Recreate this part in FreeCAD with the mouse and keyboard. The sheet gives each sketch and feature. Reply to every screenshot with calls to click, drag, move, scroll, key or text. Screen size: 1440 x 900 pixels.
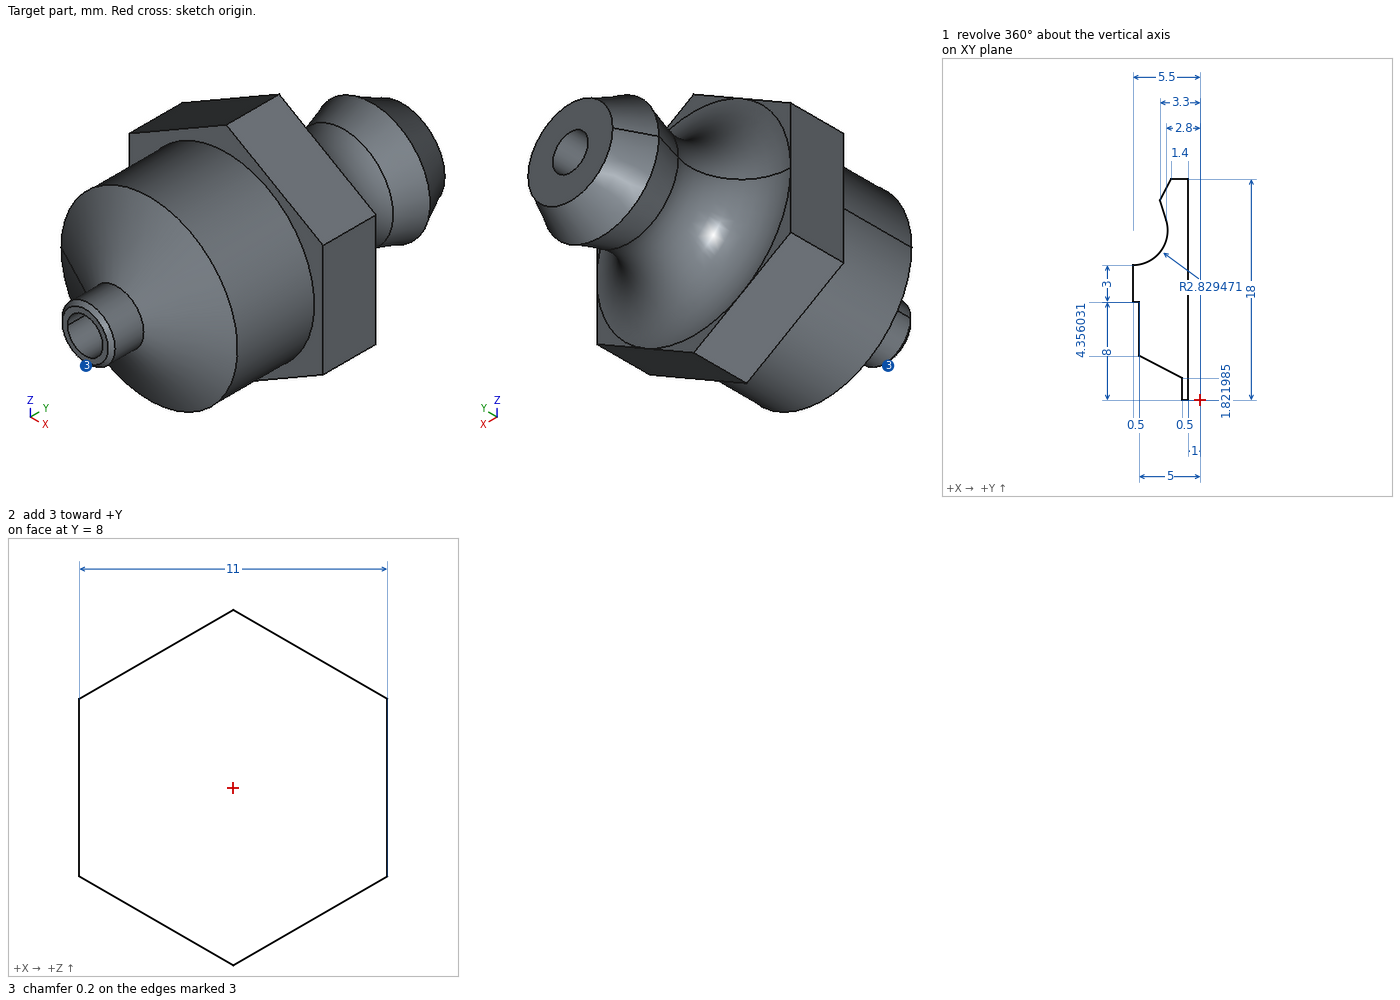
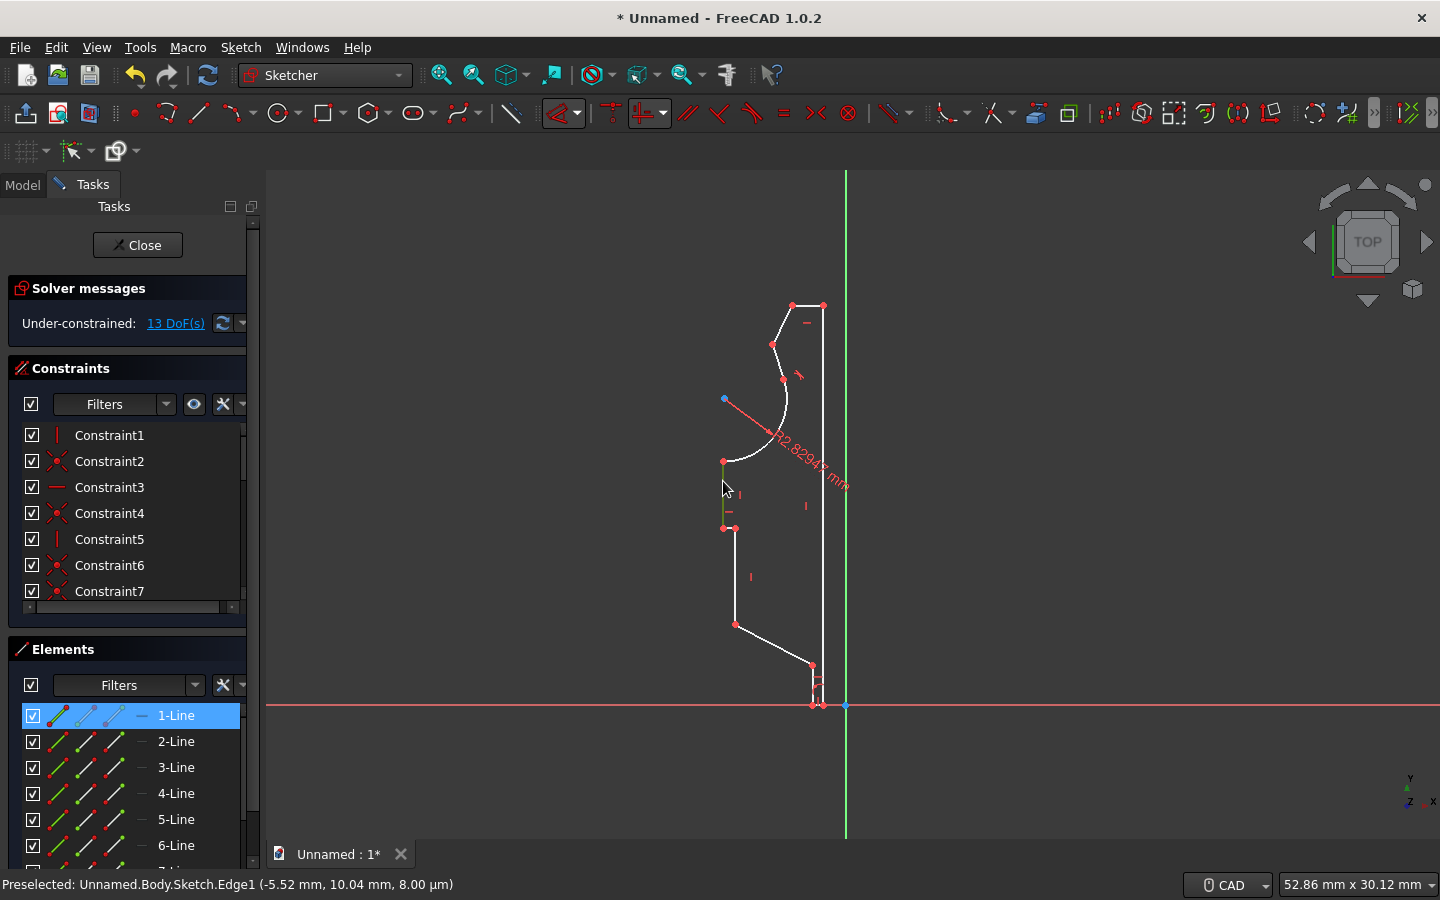
click(580, 114)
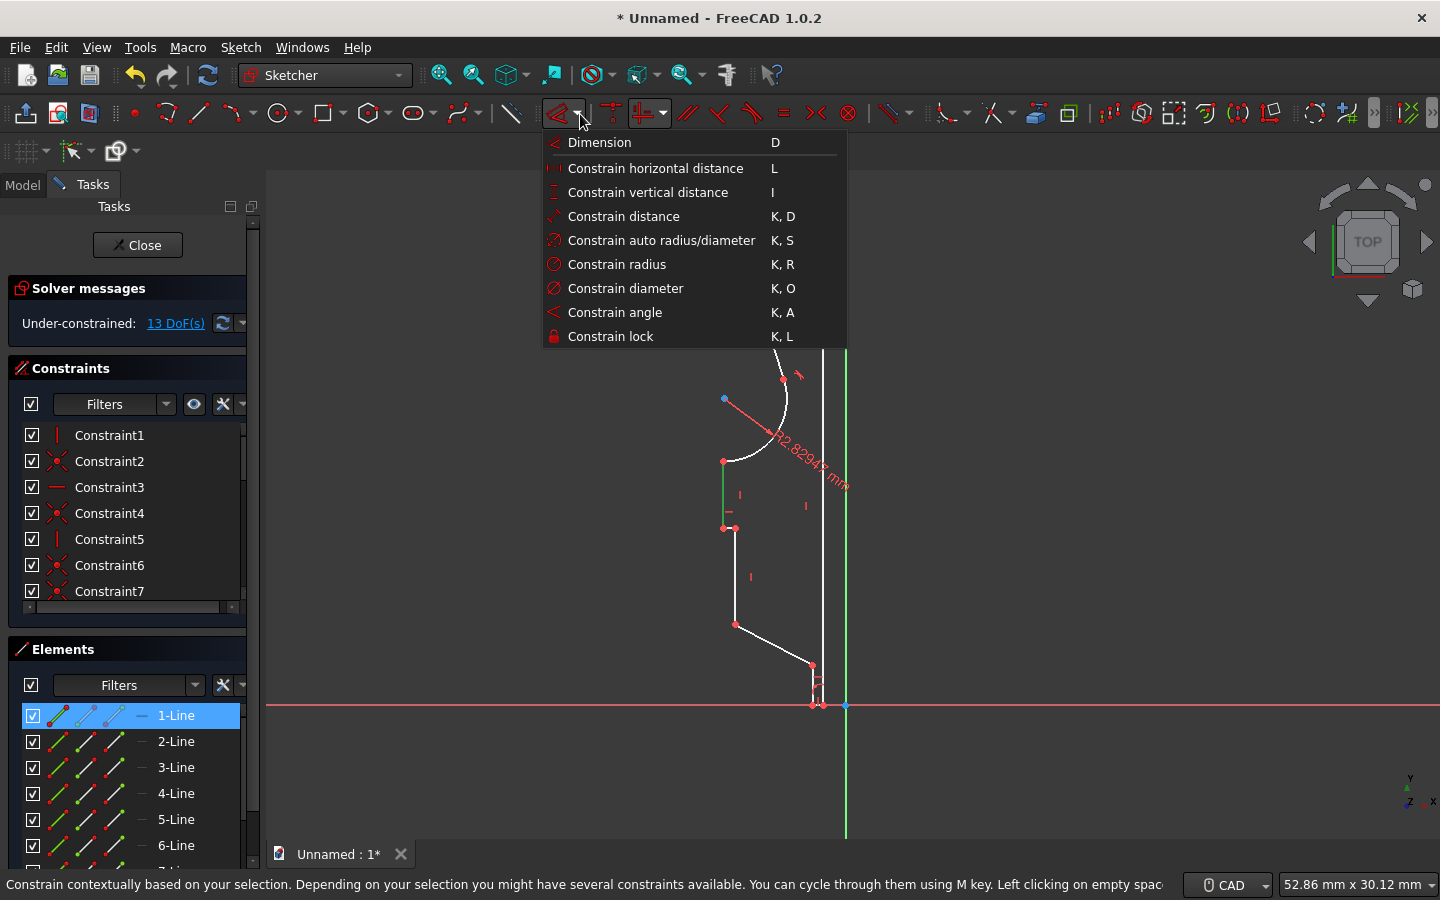
click(695, 192)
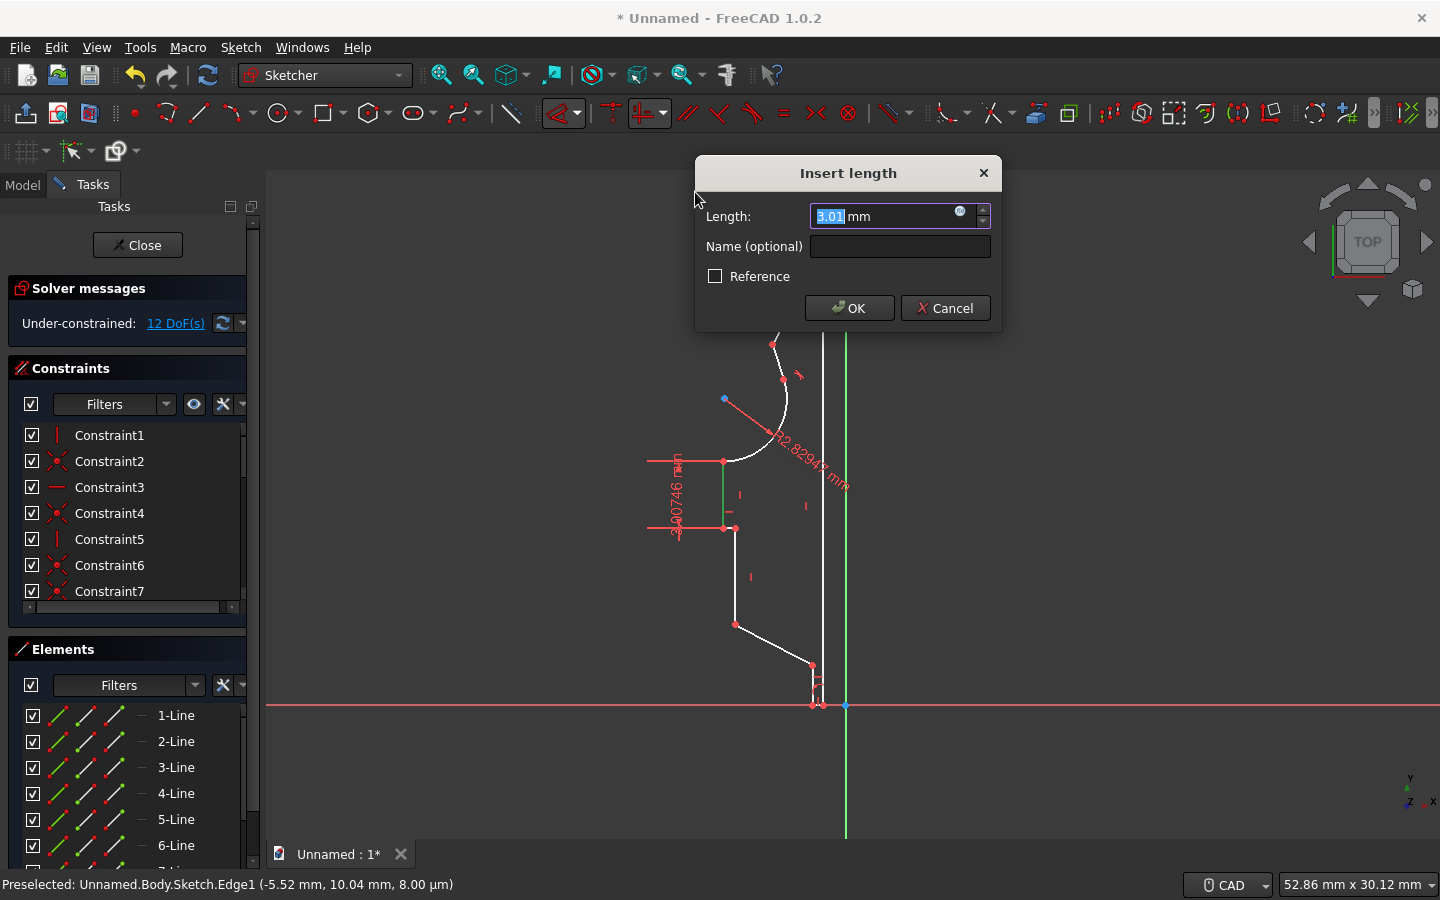
text(3)
key(Return)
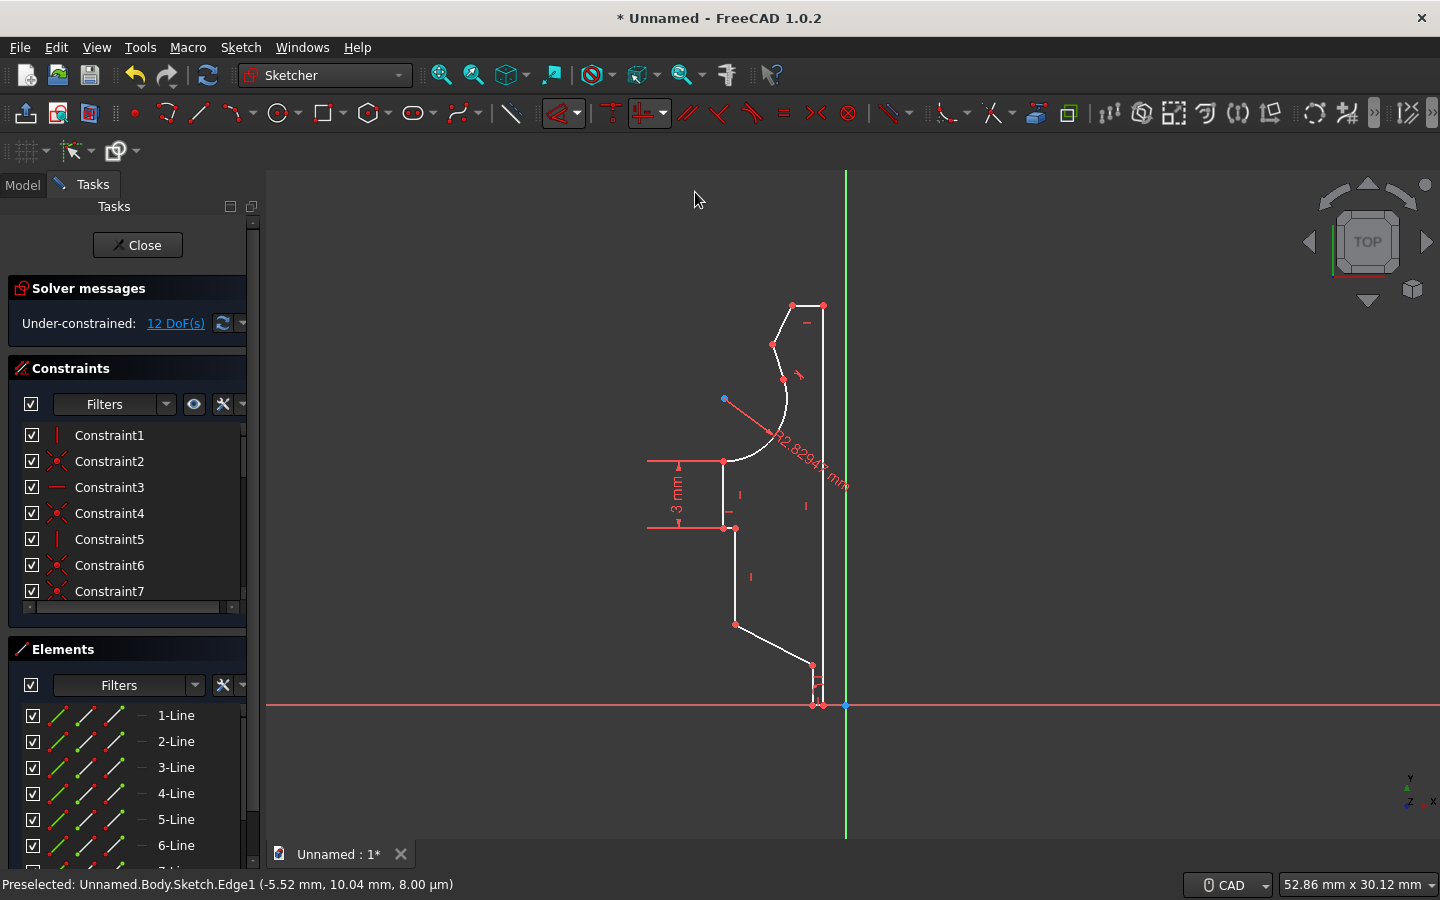
click(823, 585)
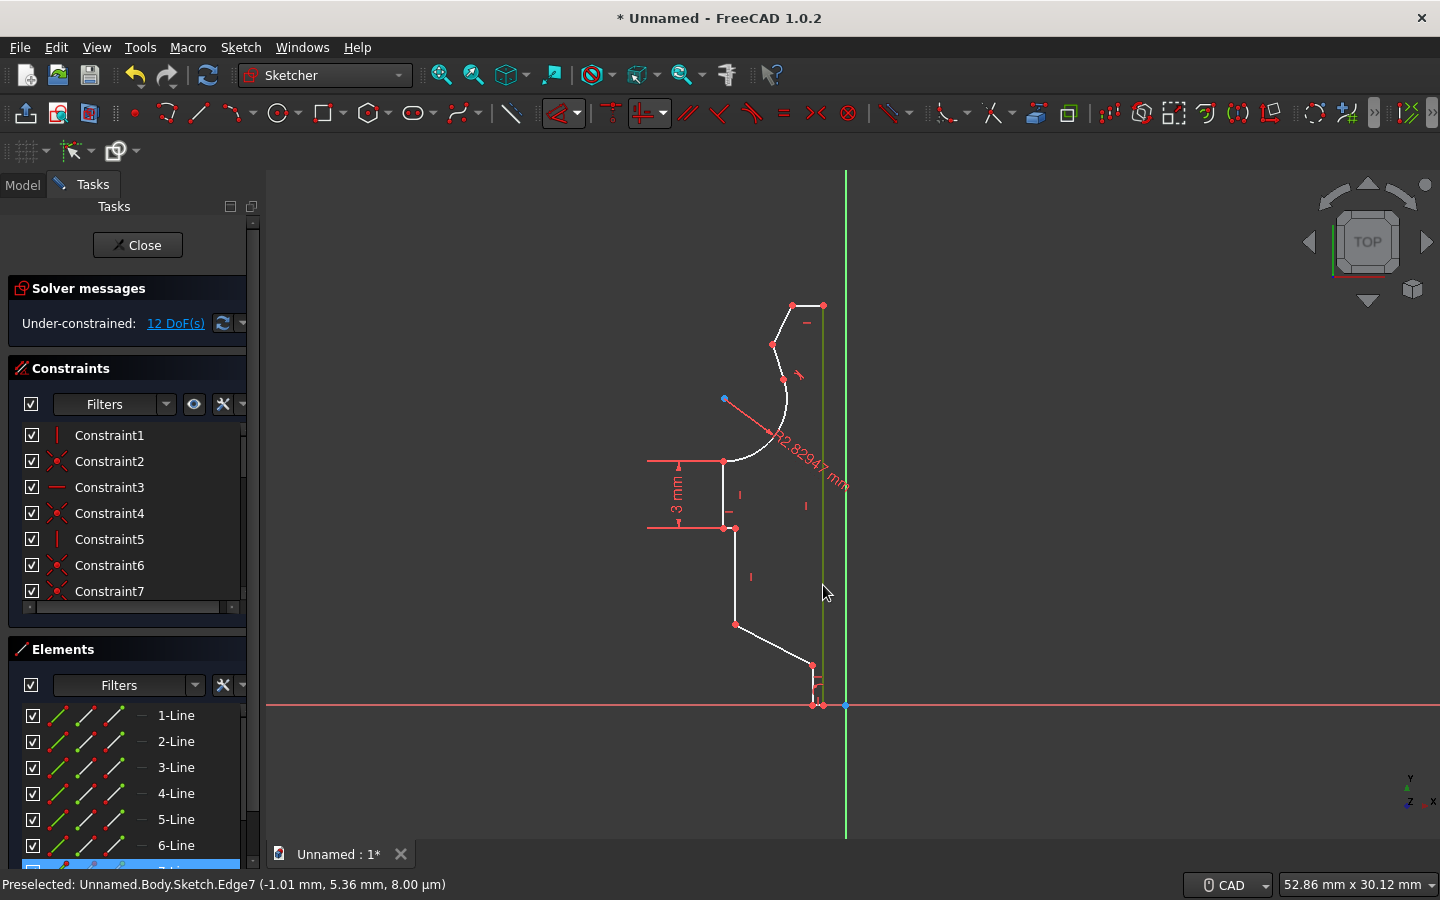
click(580, 114)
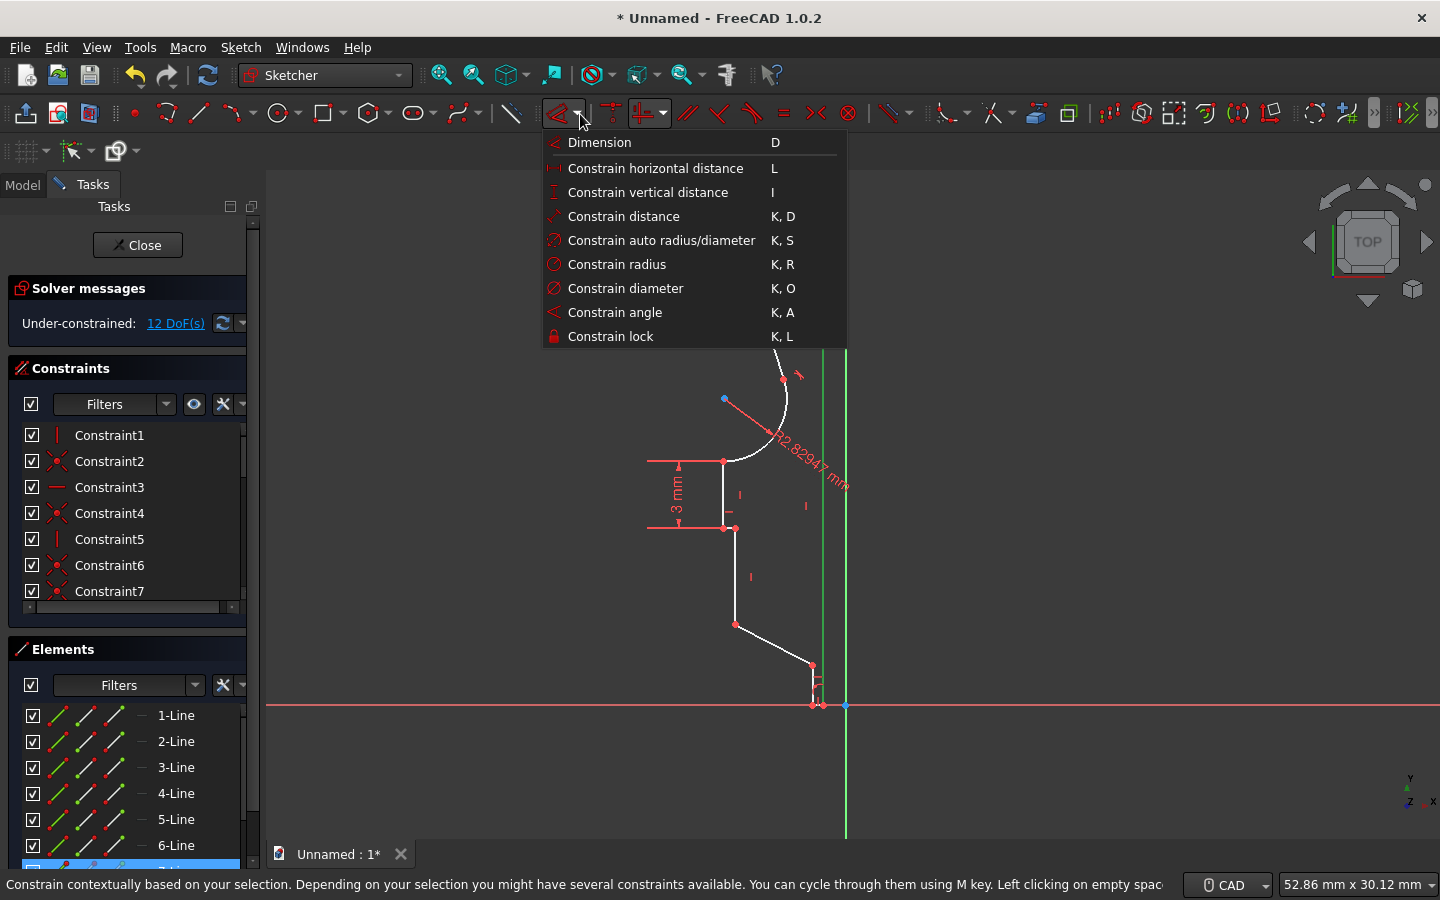
click(695, 192)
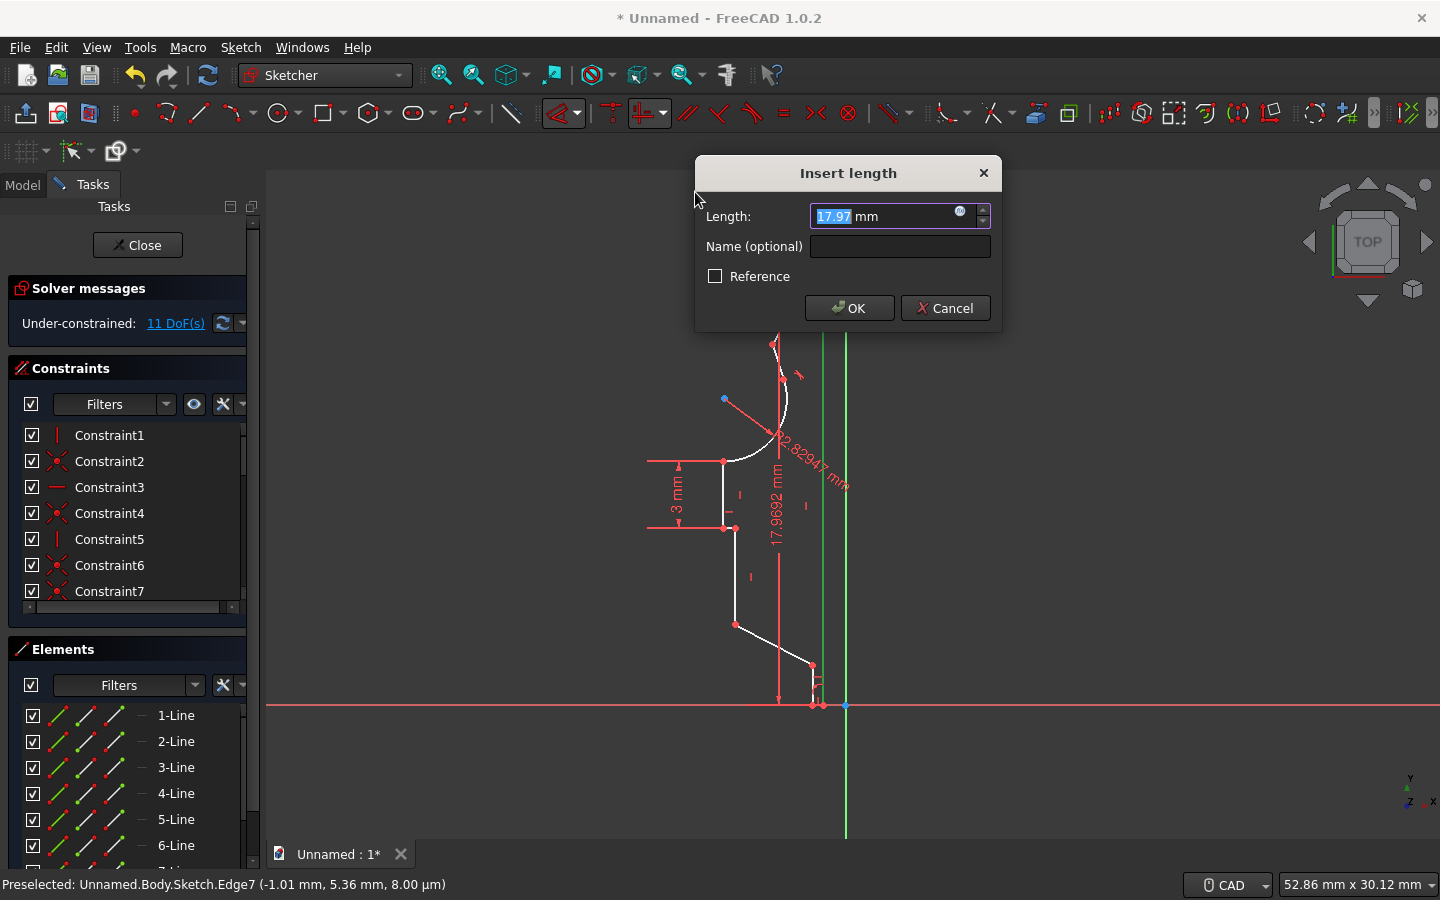
text(18)
key(Return)